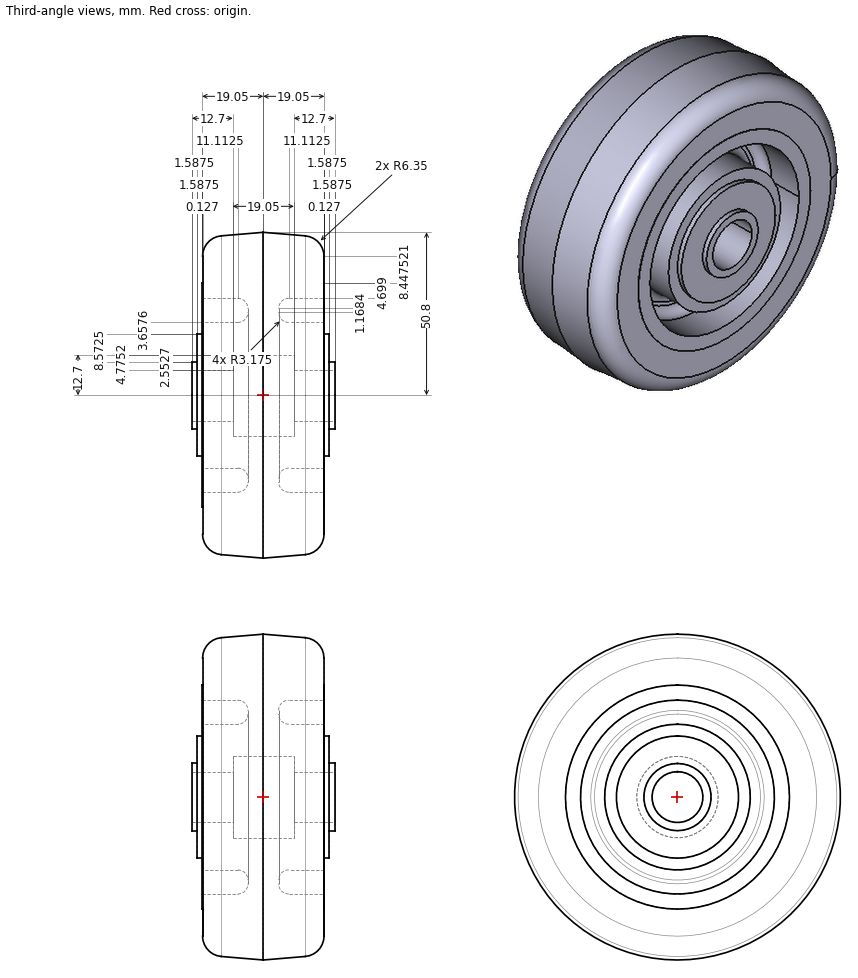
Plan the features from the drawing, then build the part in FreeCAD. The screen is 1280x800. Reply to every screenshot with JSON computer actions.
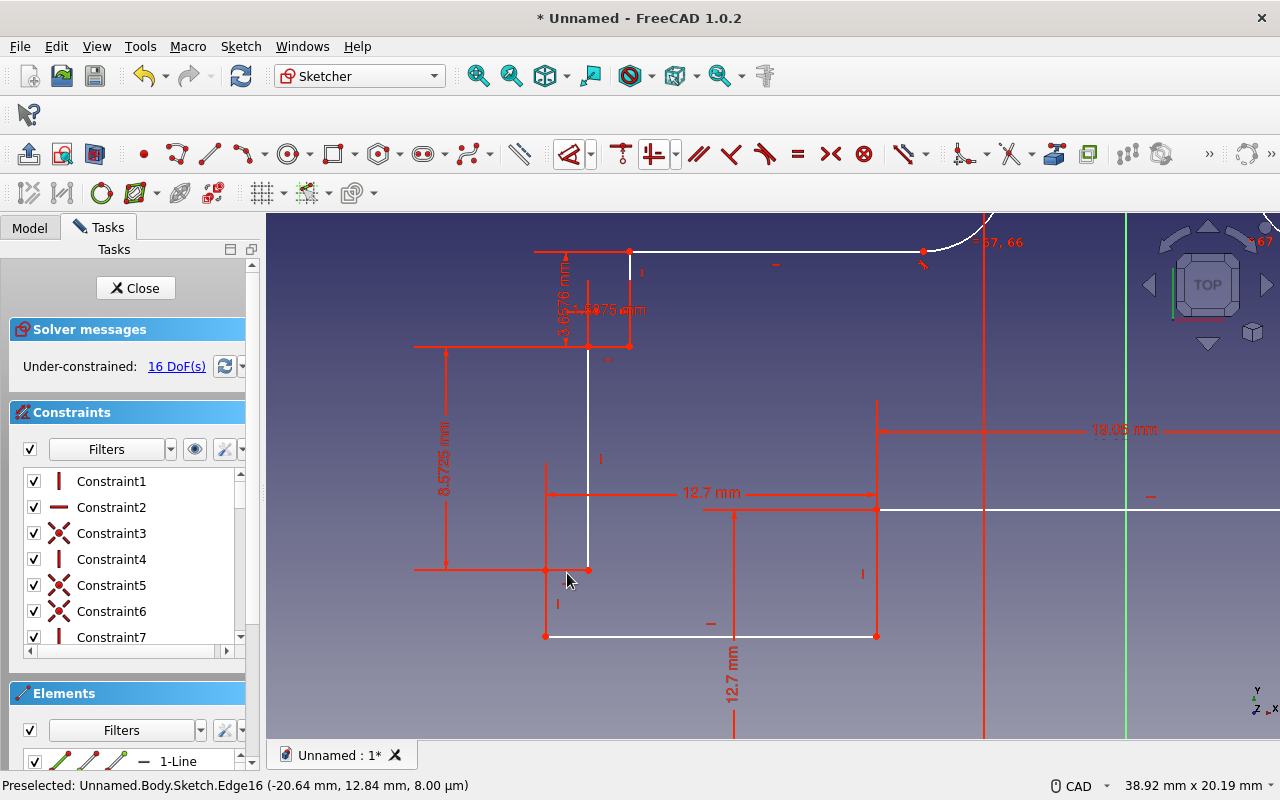
{"action": "left_click", "coordinate": [567, 570]}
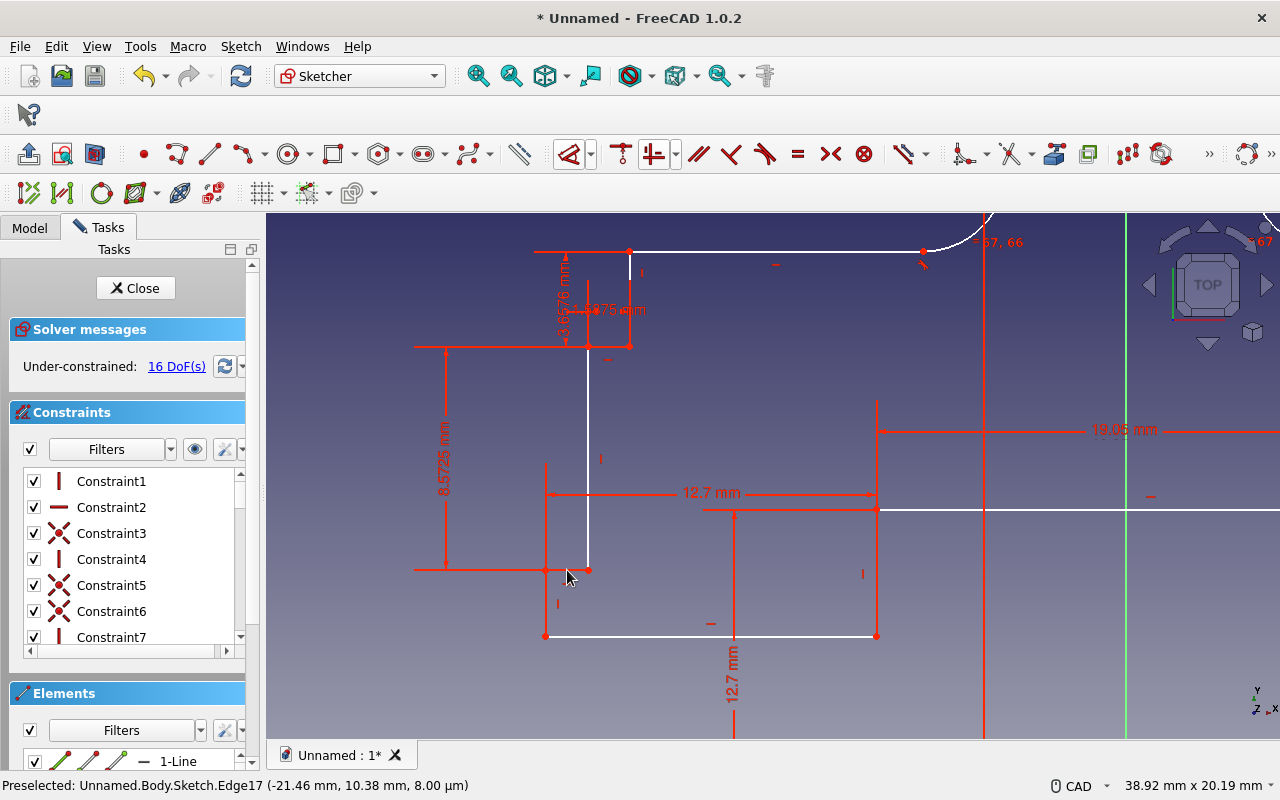
{"action": "left_click", "coordinate": [590, 154]}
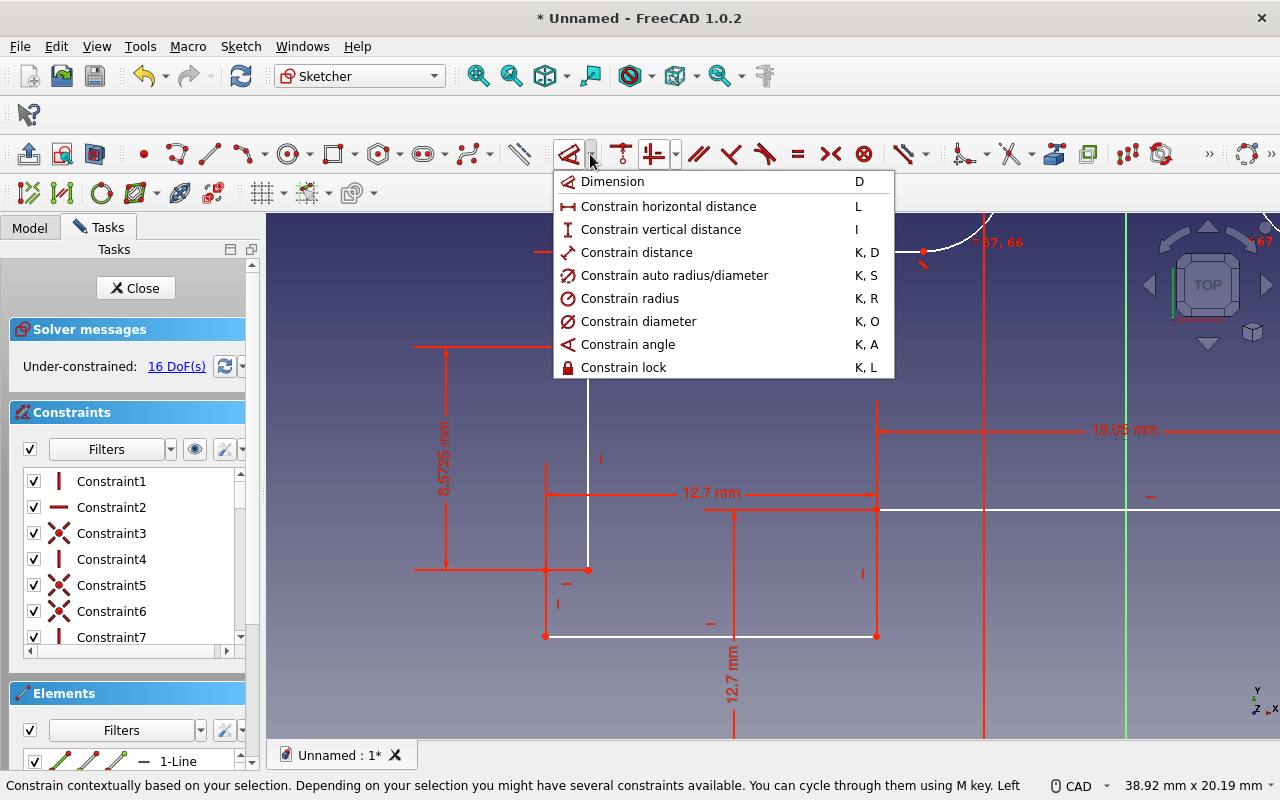
{"action": "left_click", "coordinate": [724, 206]}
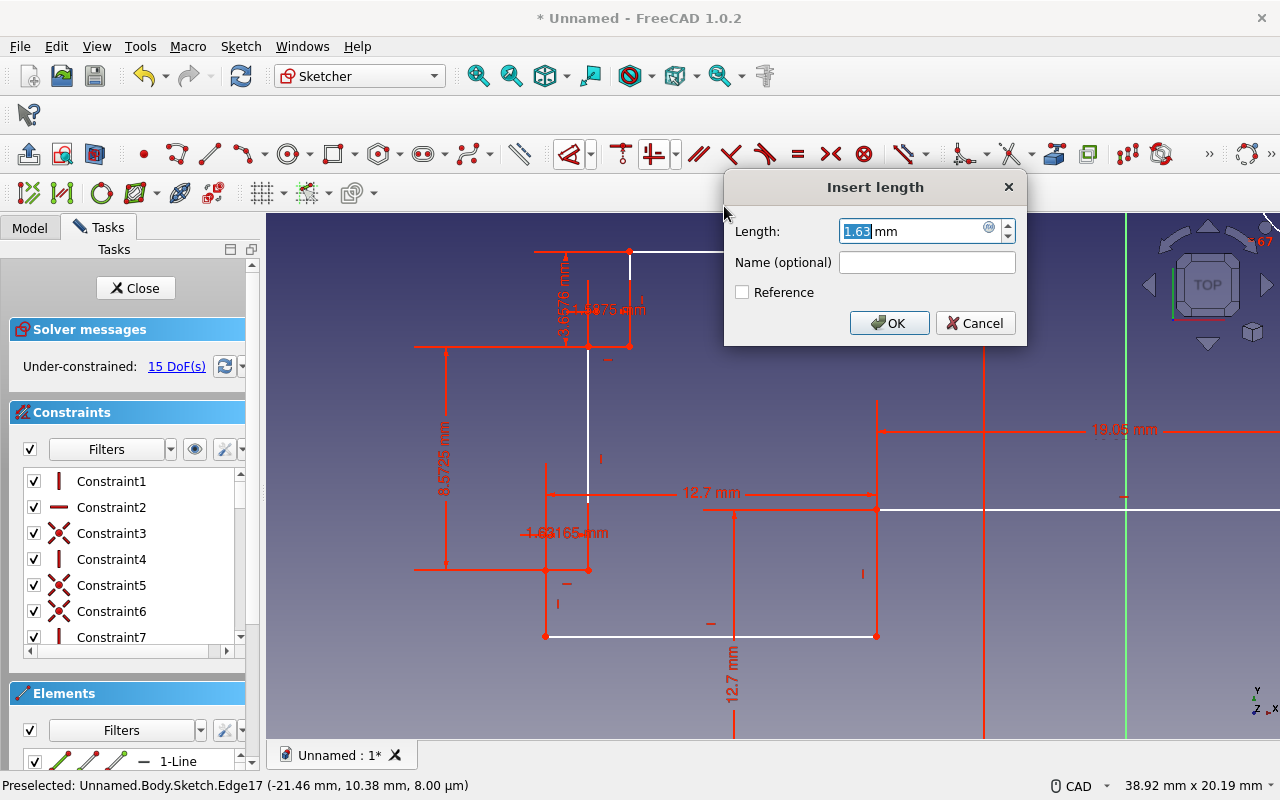
{"action": "type", "text": "1.5875"}
{"action": "key", "text": "Return"}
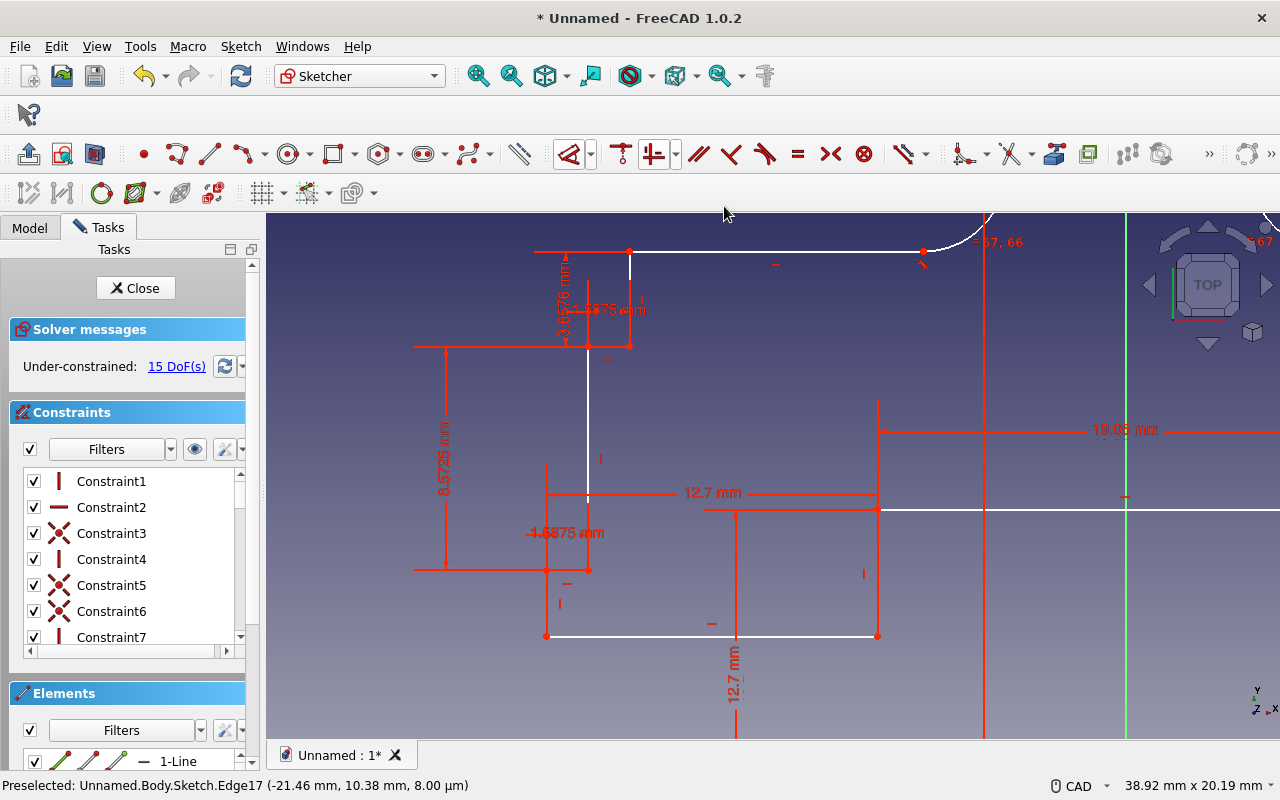
{"action": "left_click", "coordinate": [547, 590]}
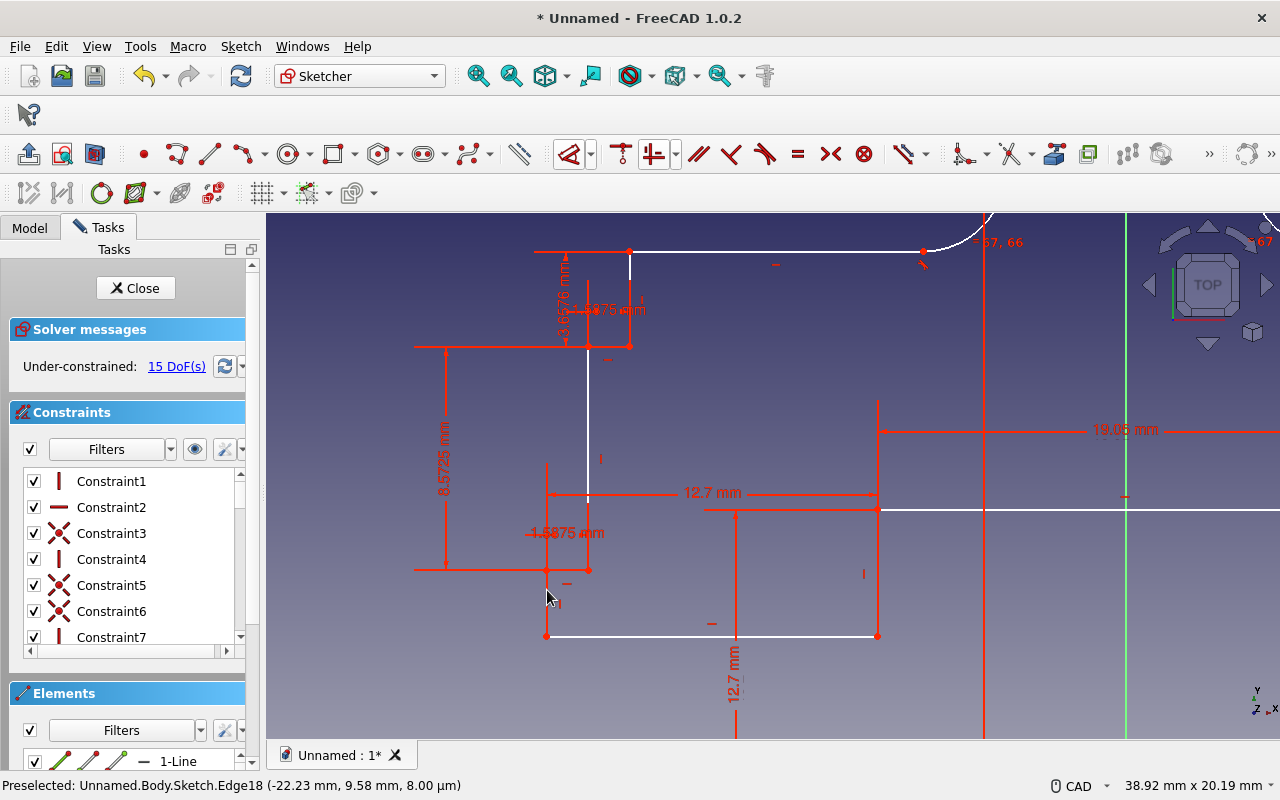
{"action": "left_click", "coordinate": [590, 154]}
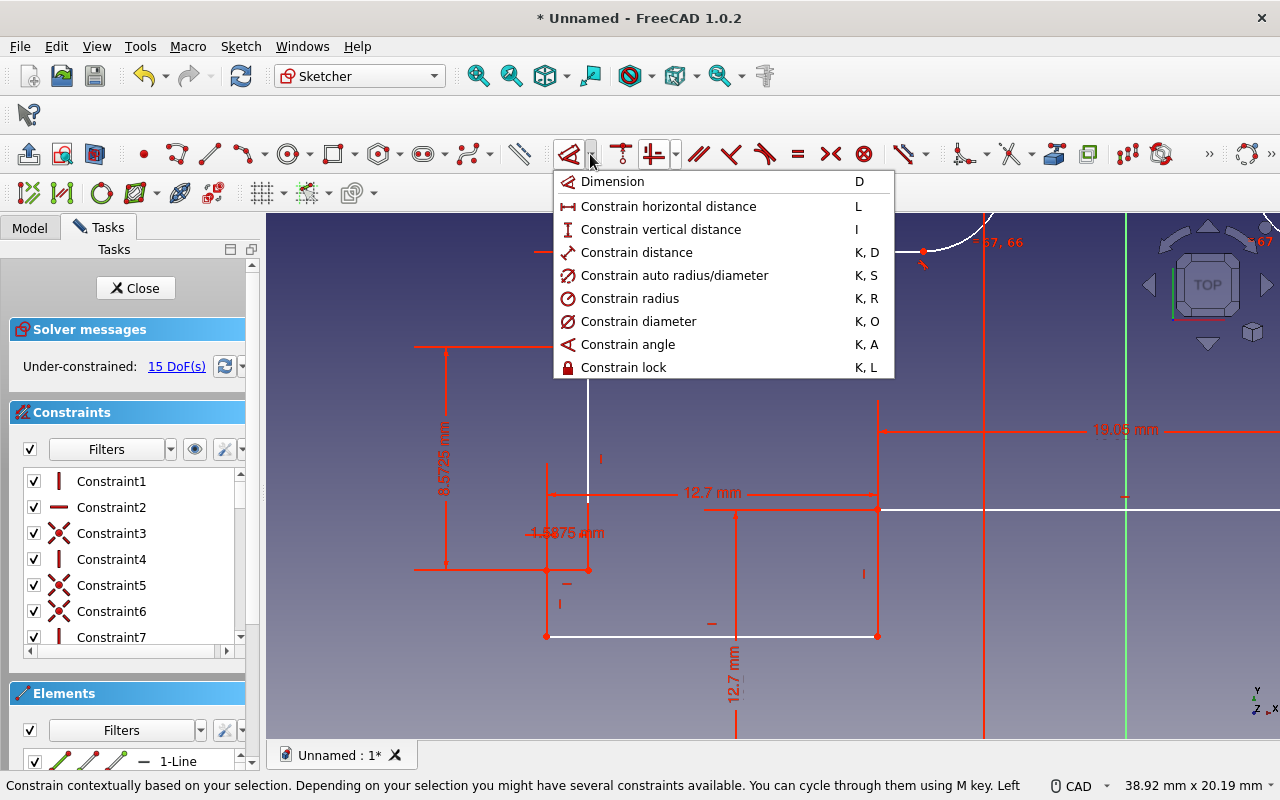
{"action": "left_click", "coordinate": [724, 230]}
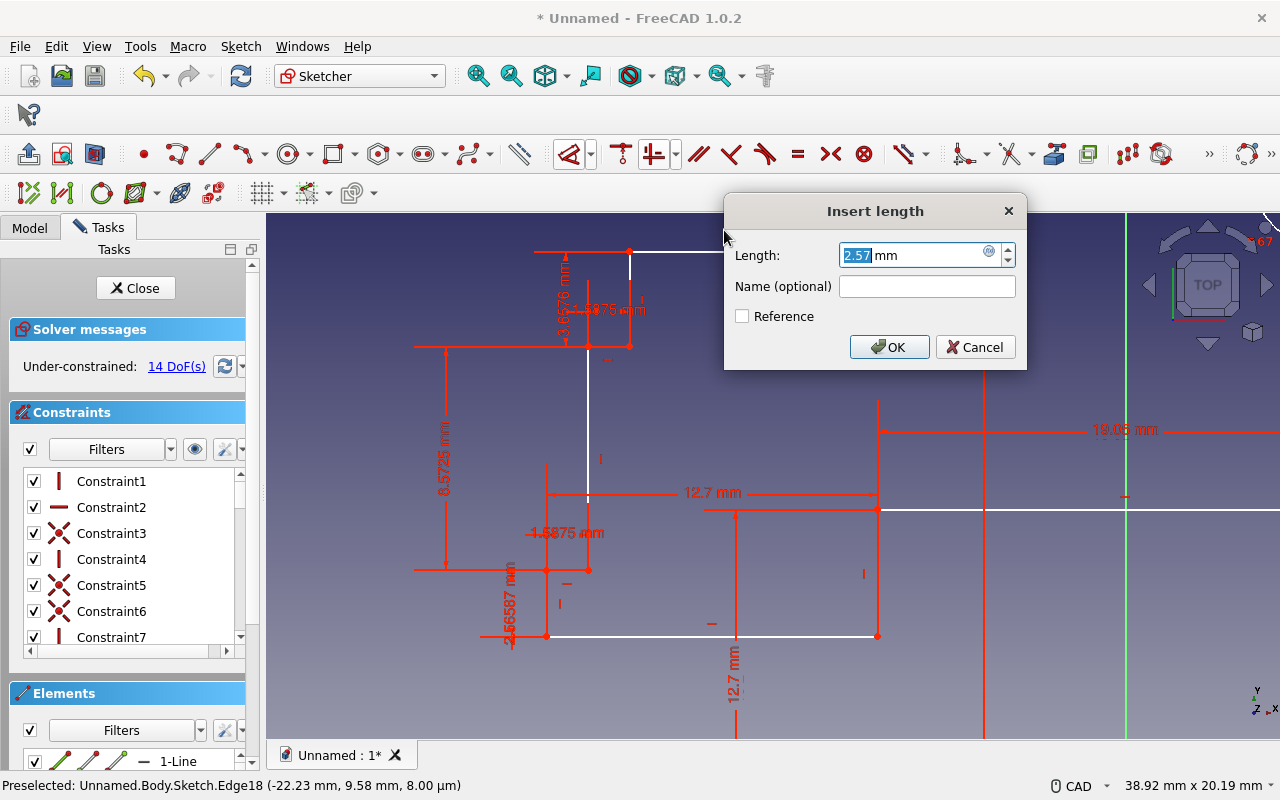
{"action": "type", "text": "2.5527"}
{"action": "key", "text": "Return"}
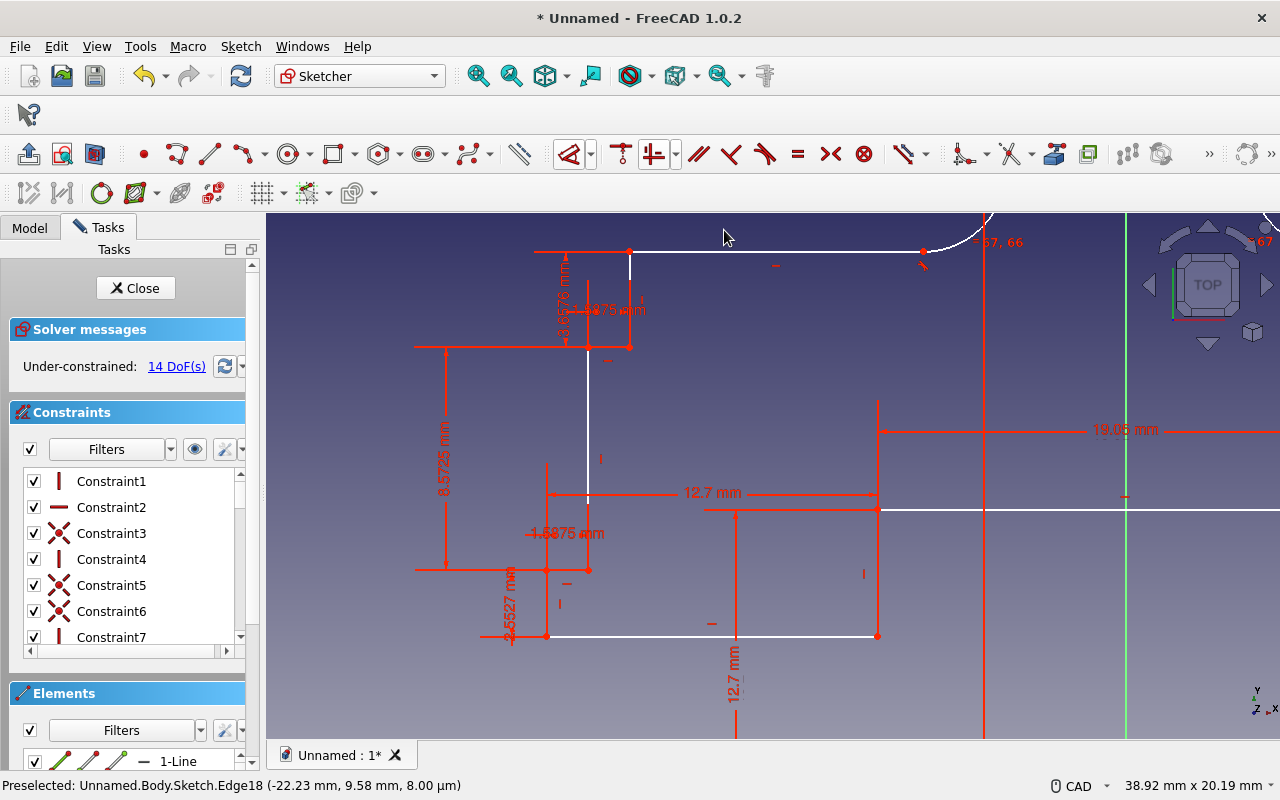
{"action": "left_click", "coordinate": [878, 599]}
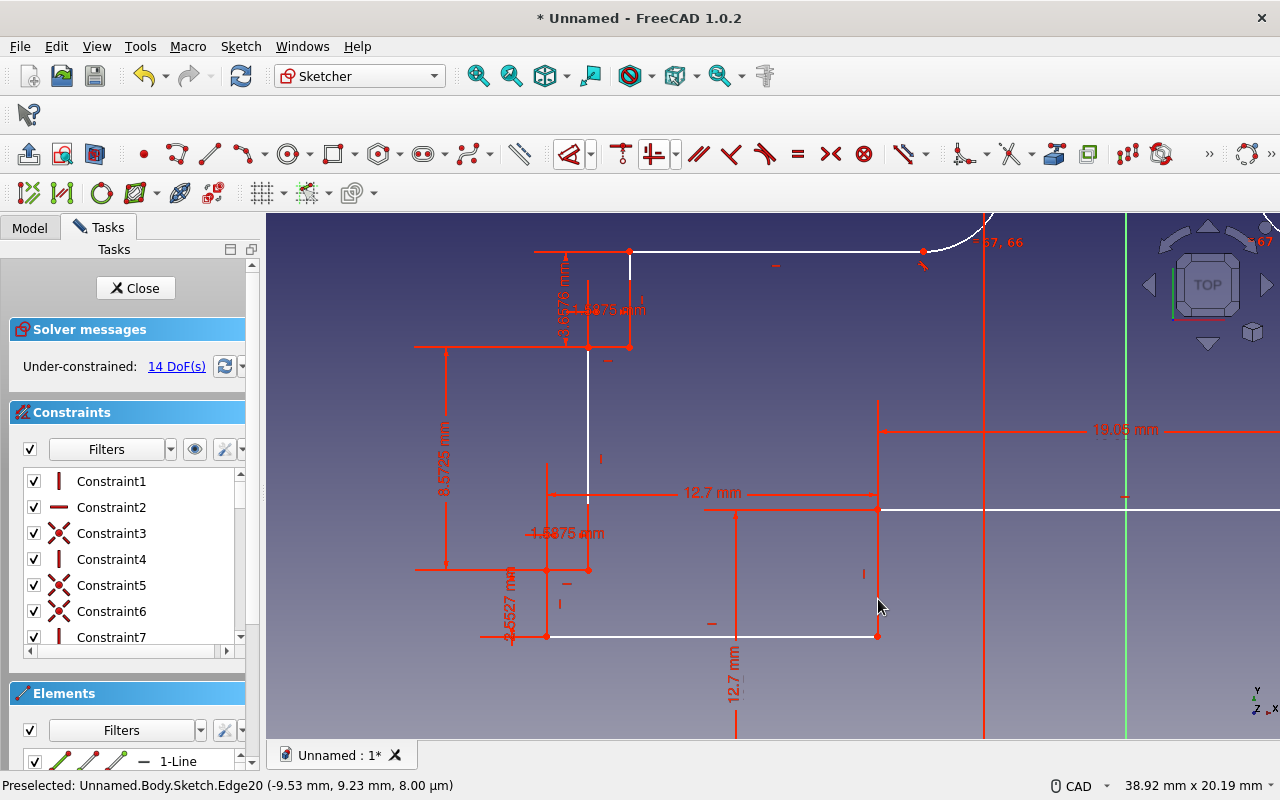
{"action": "left_click", "coordinate": [590, 154]}